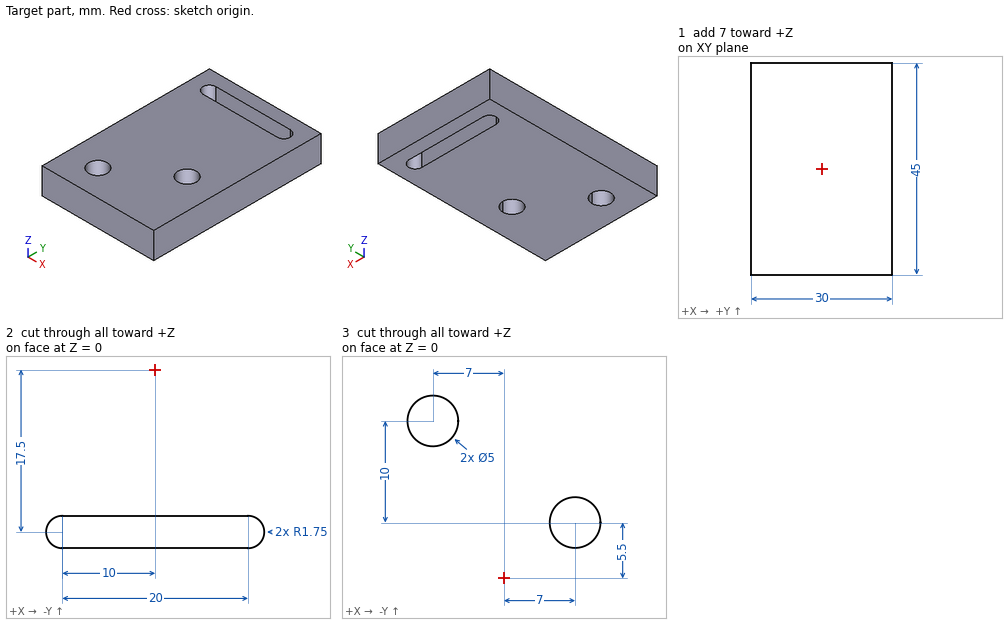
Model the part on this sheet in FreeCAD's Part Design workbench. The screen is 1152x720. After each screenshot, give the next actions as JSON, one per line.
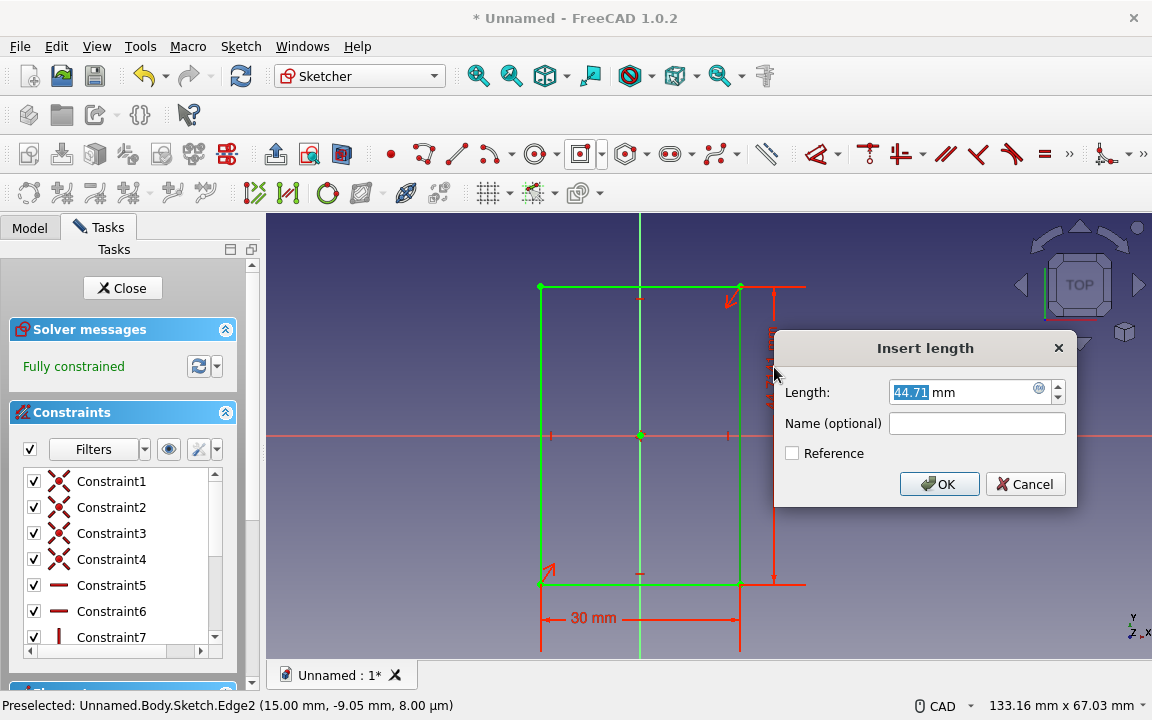
{"action": "type", "text": "45"}
{"action": "key", "text": "Return"}
{"action": "key", "text": "Escape"}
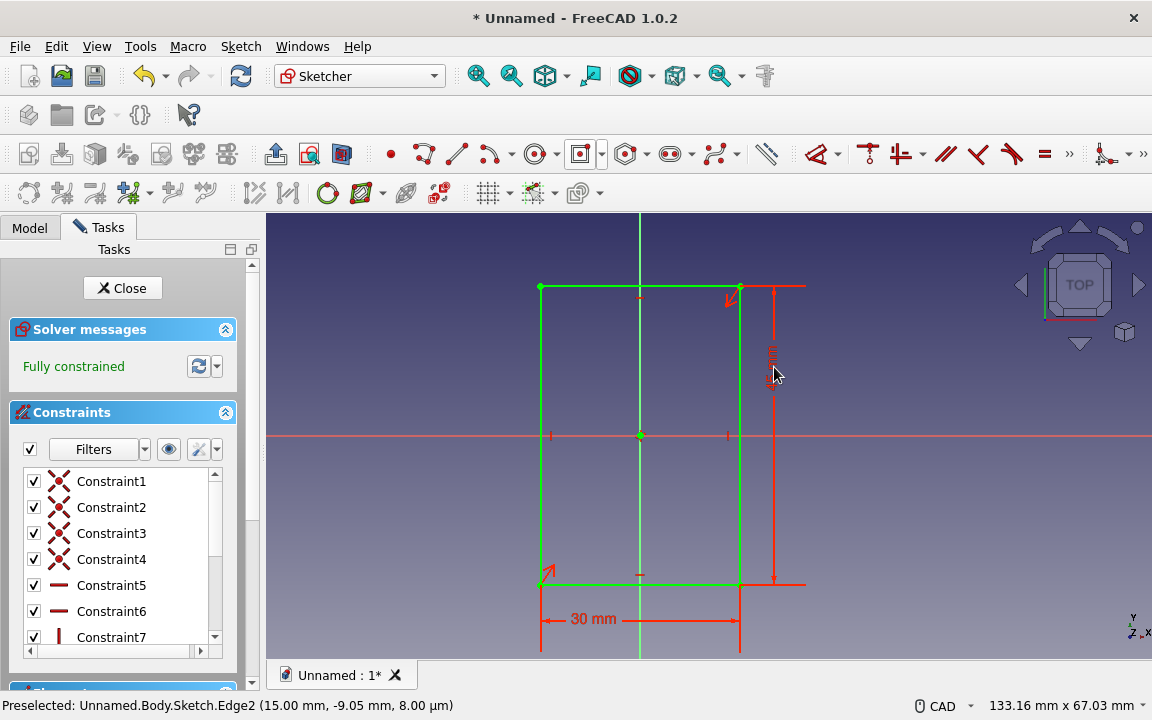
{"action": "left_click", "coordinate": [123, 288]}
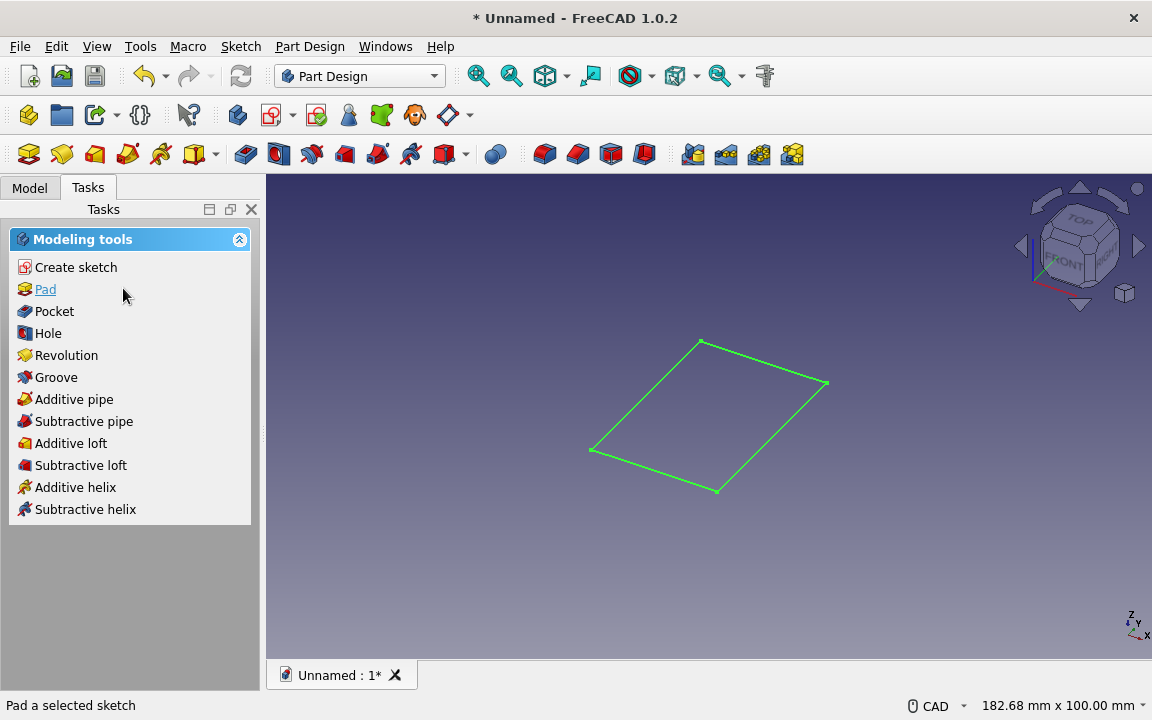
{"action": "left_click", "coordinate": [29, 154]}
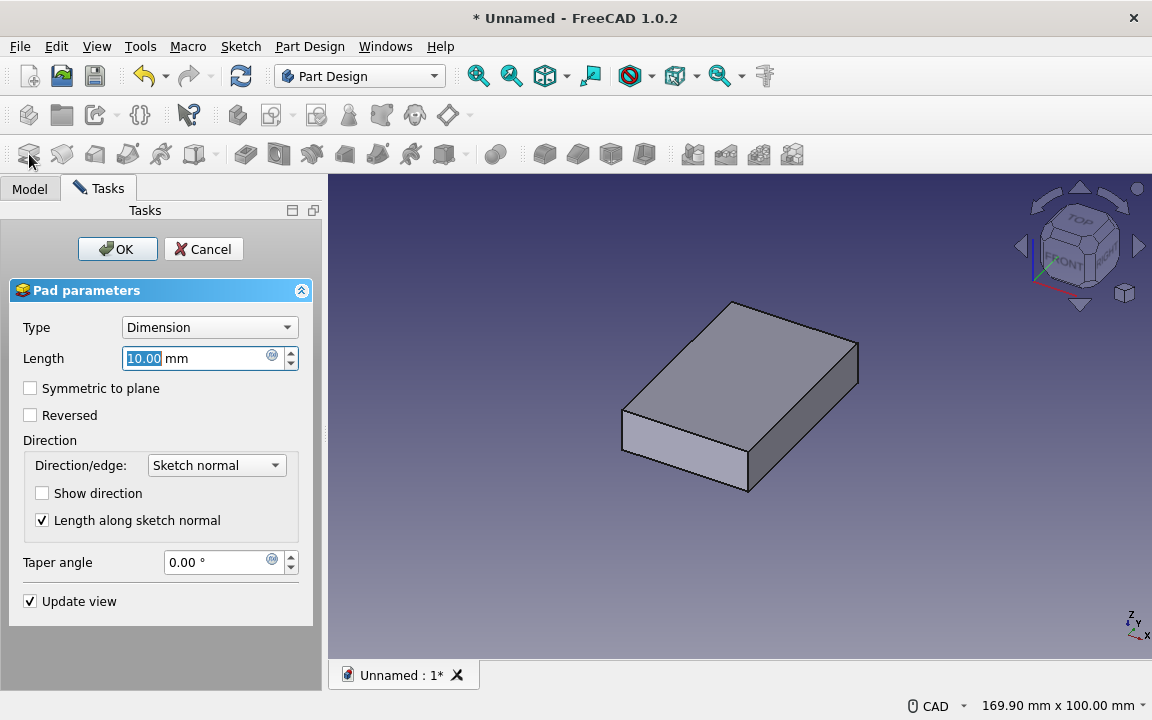
{"action": "type", "text": "7"}
{"action": "key", "text": "Tab"}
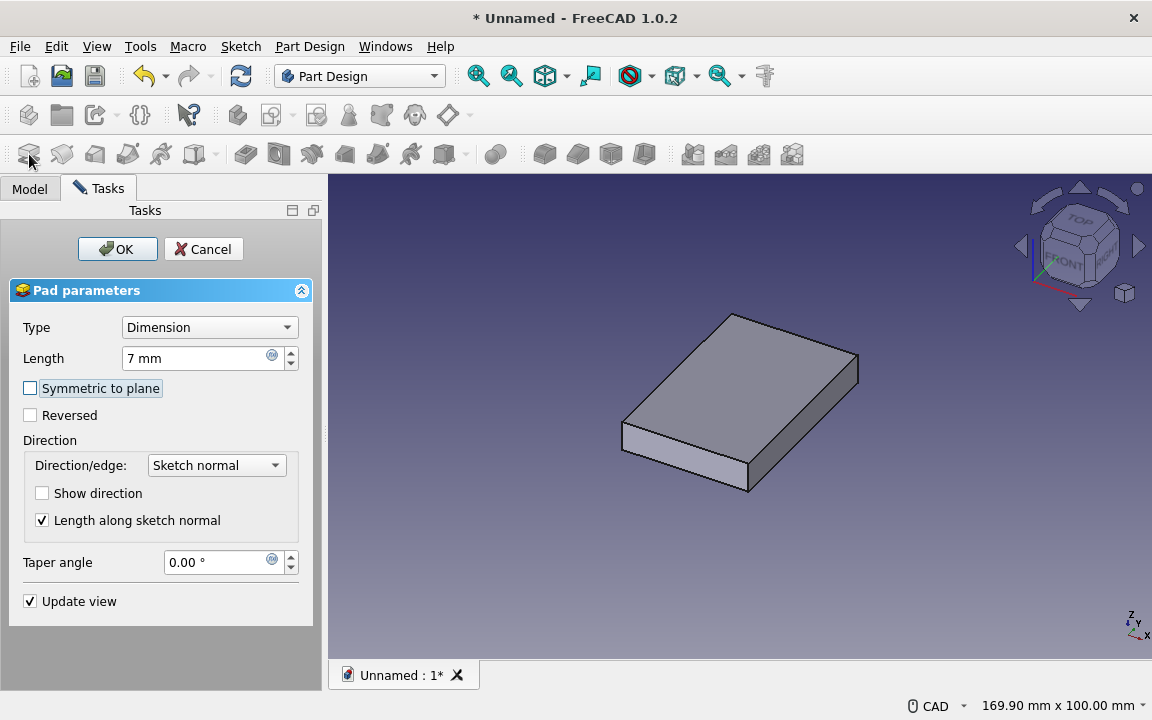
{"action": "left_click", "coordinate": [118, 249]}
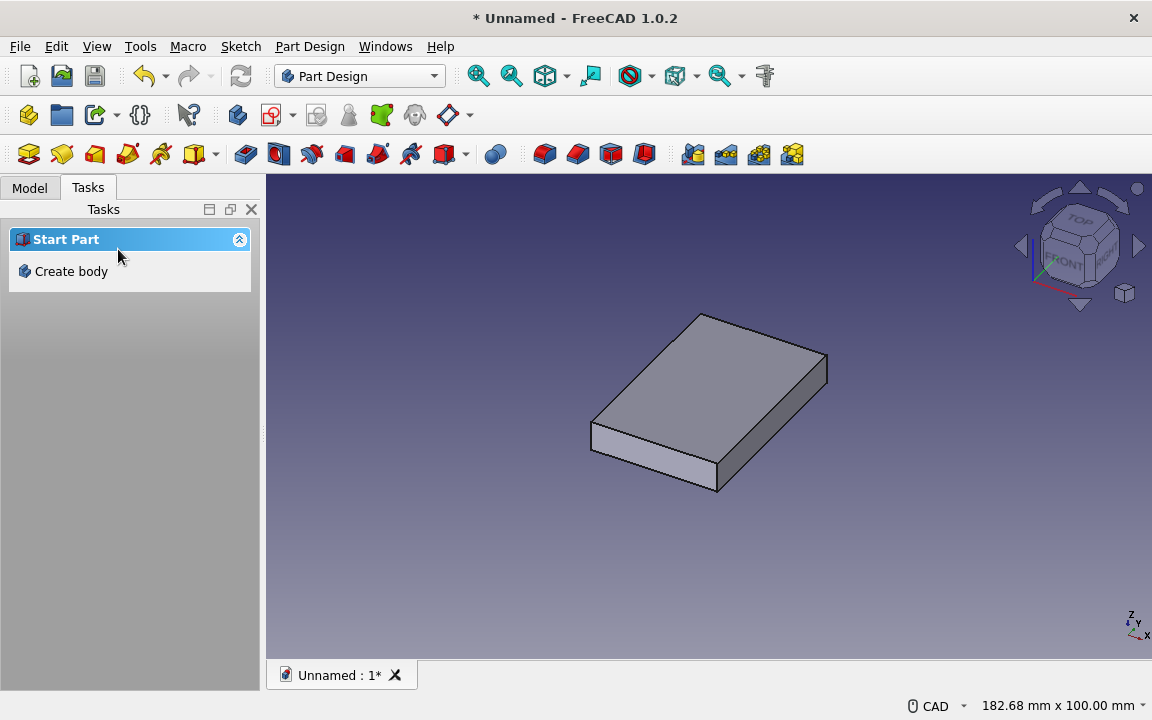
{"action": "left_click", "coordinate": [479, 76]}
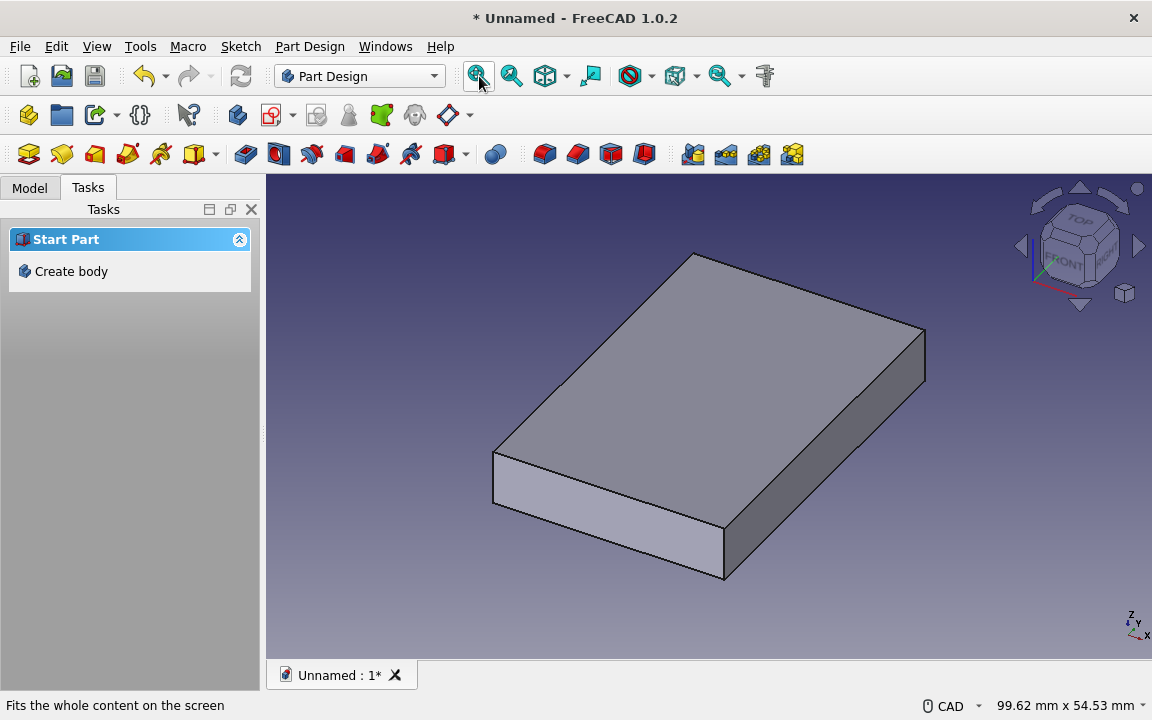
{"action": "key", "text": "5"}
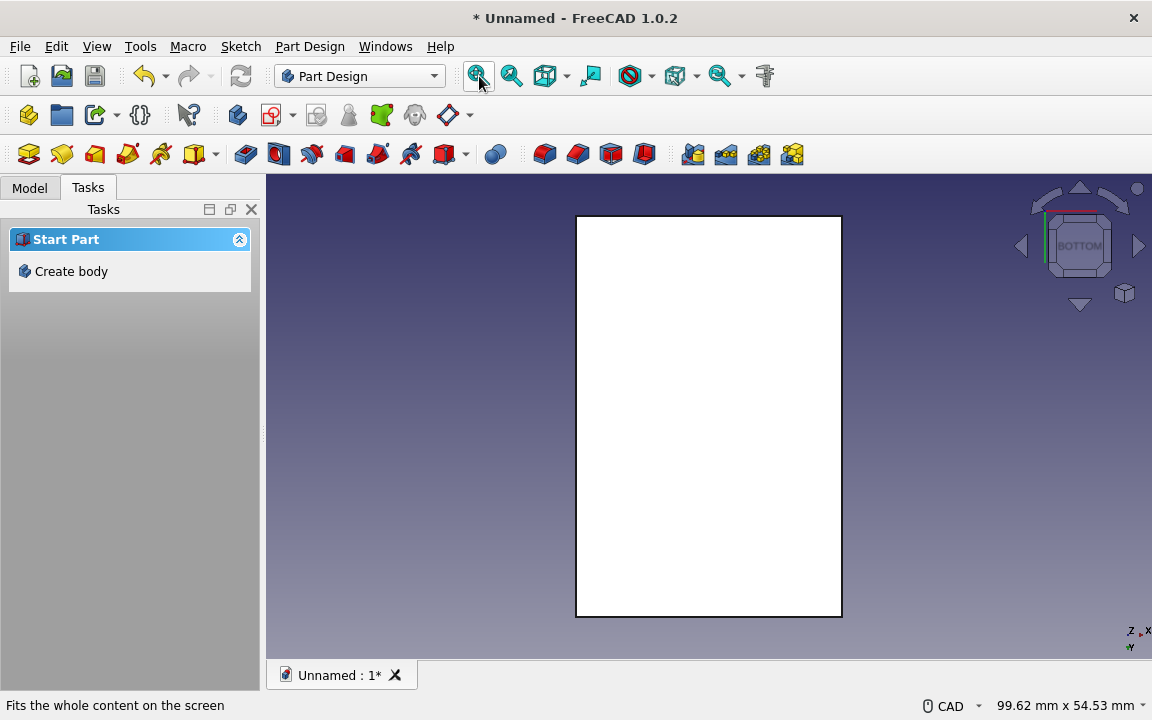
{"action": "left_click", "coordinate": [709, 473]}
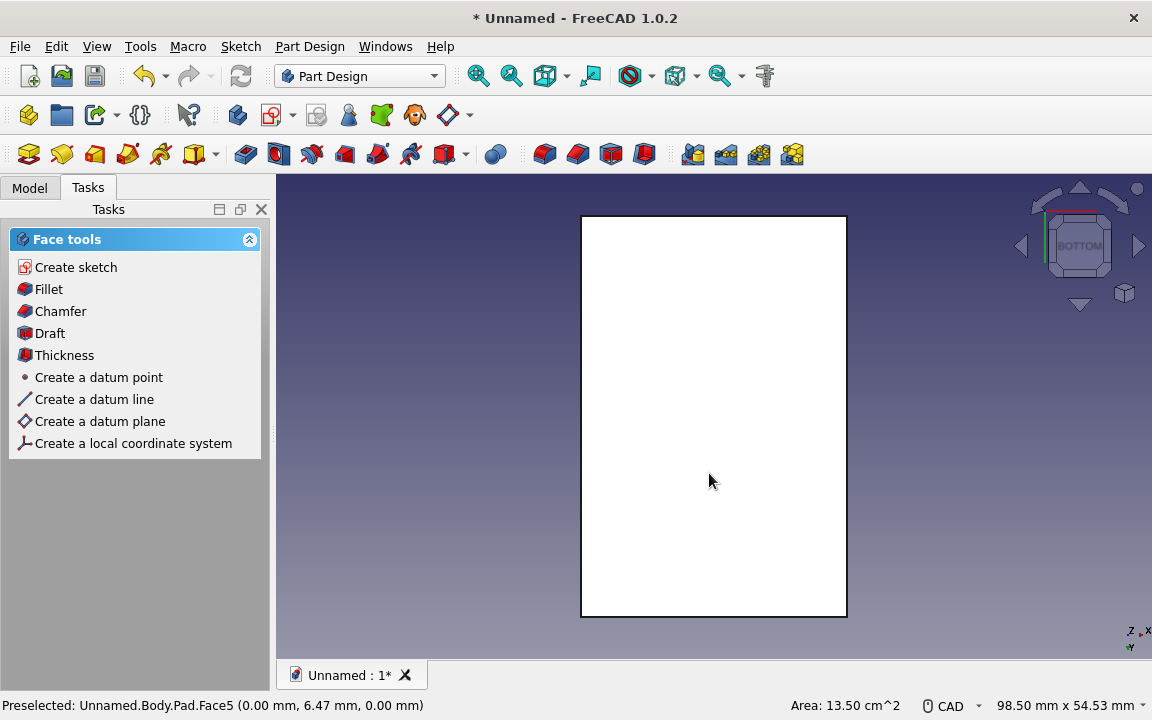
{"action": "left_click", "coordinate": [270, 116]}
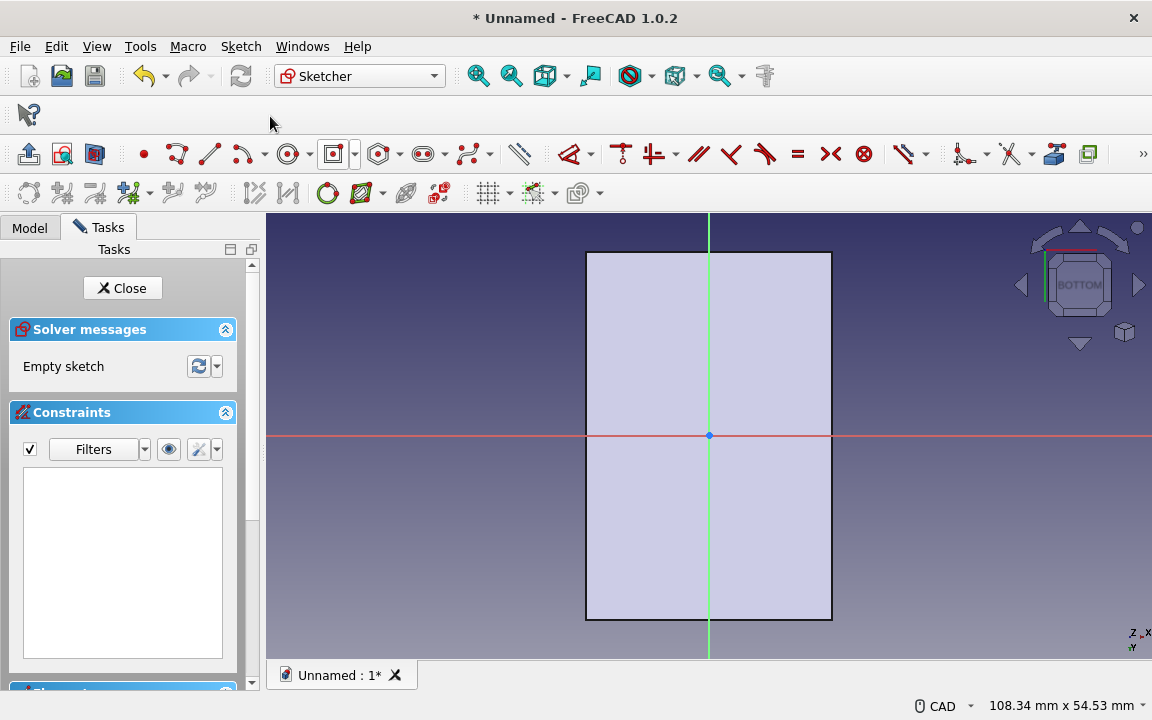
{"action": "scroll", "coordinate": [792, 610], "scroll_direction": "up", "scroll_amount": 3}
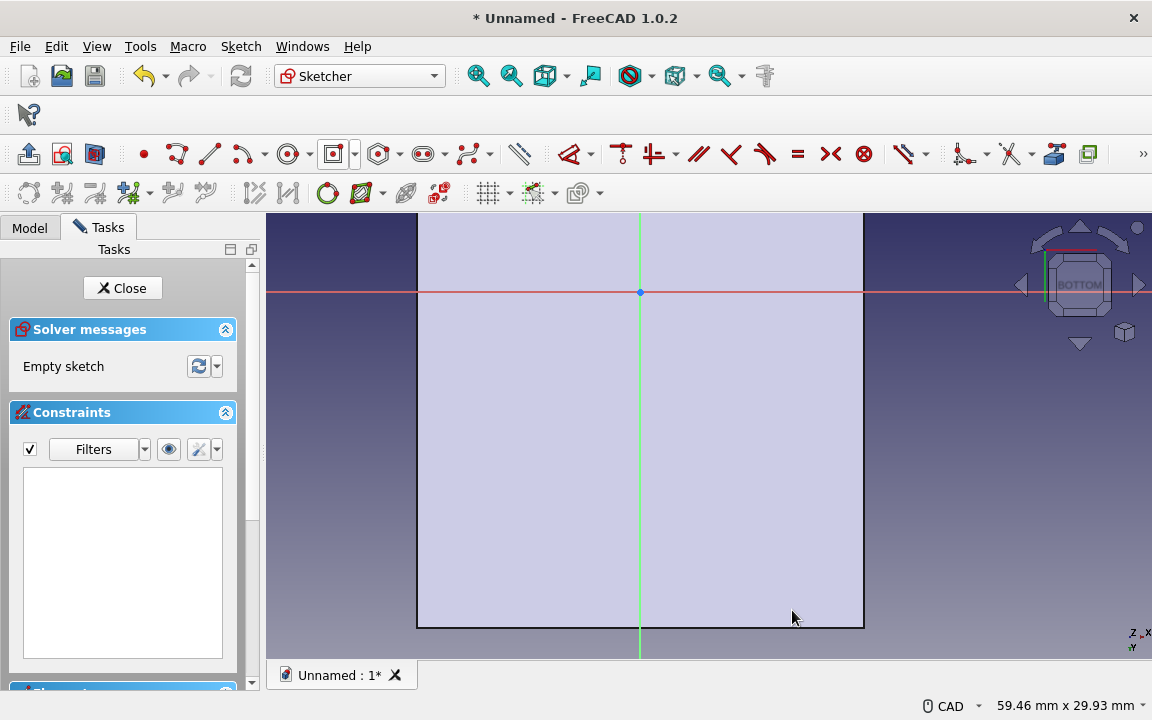
{"action": "left_click", "coordinate": [422, 154]}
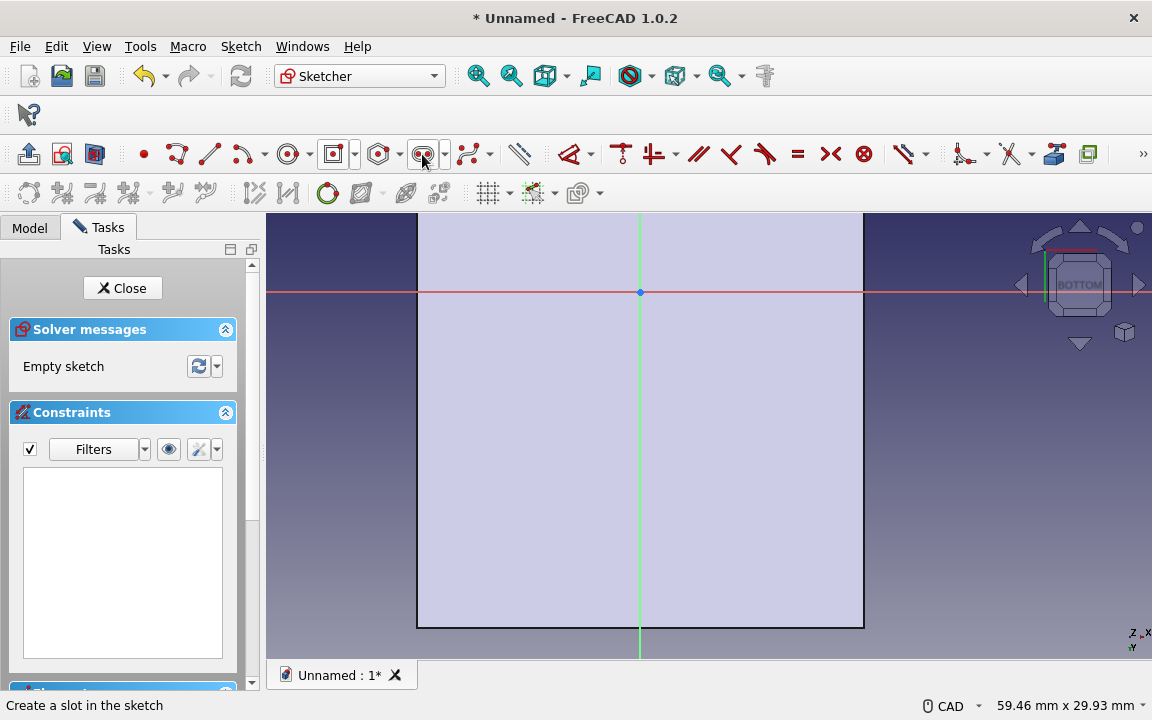
{"action": "left_click", "coordinate": [491, 553]}